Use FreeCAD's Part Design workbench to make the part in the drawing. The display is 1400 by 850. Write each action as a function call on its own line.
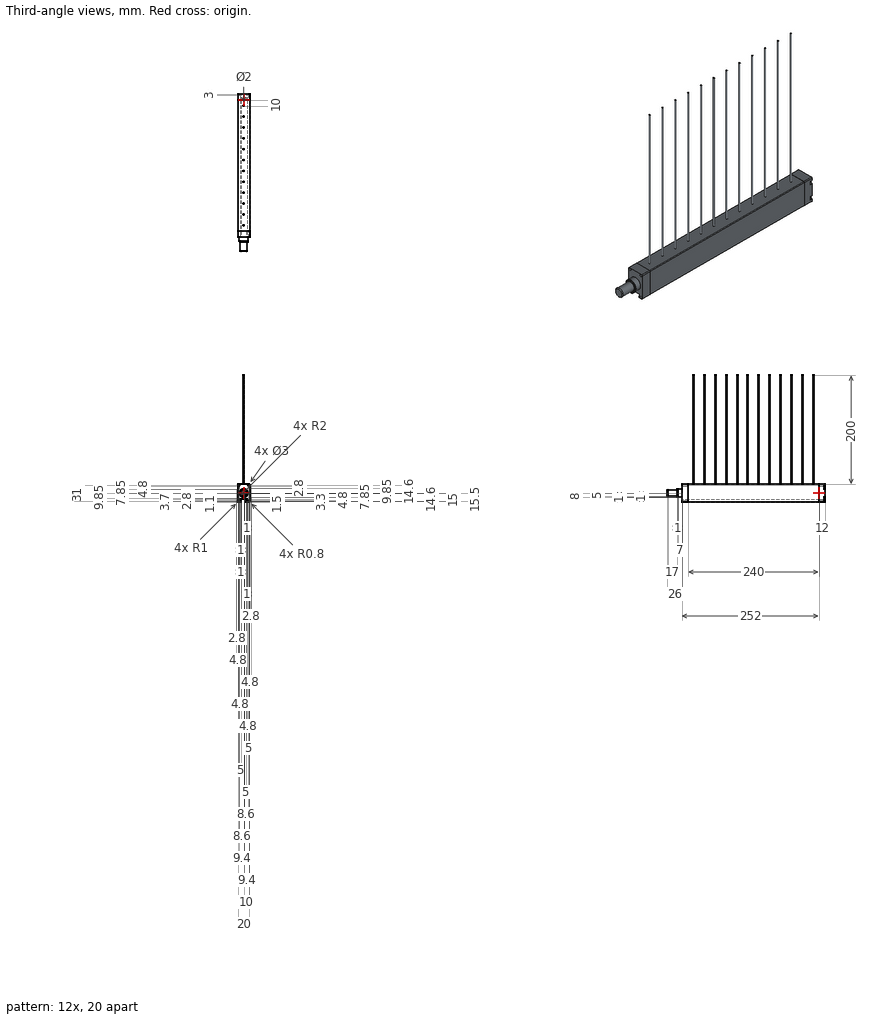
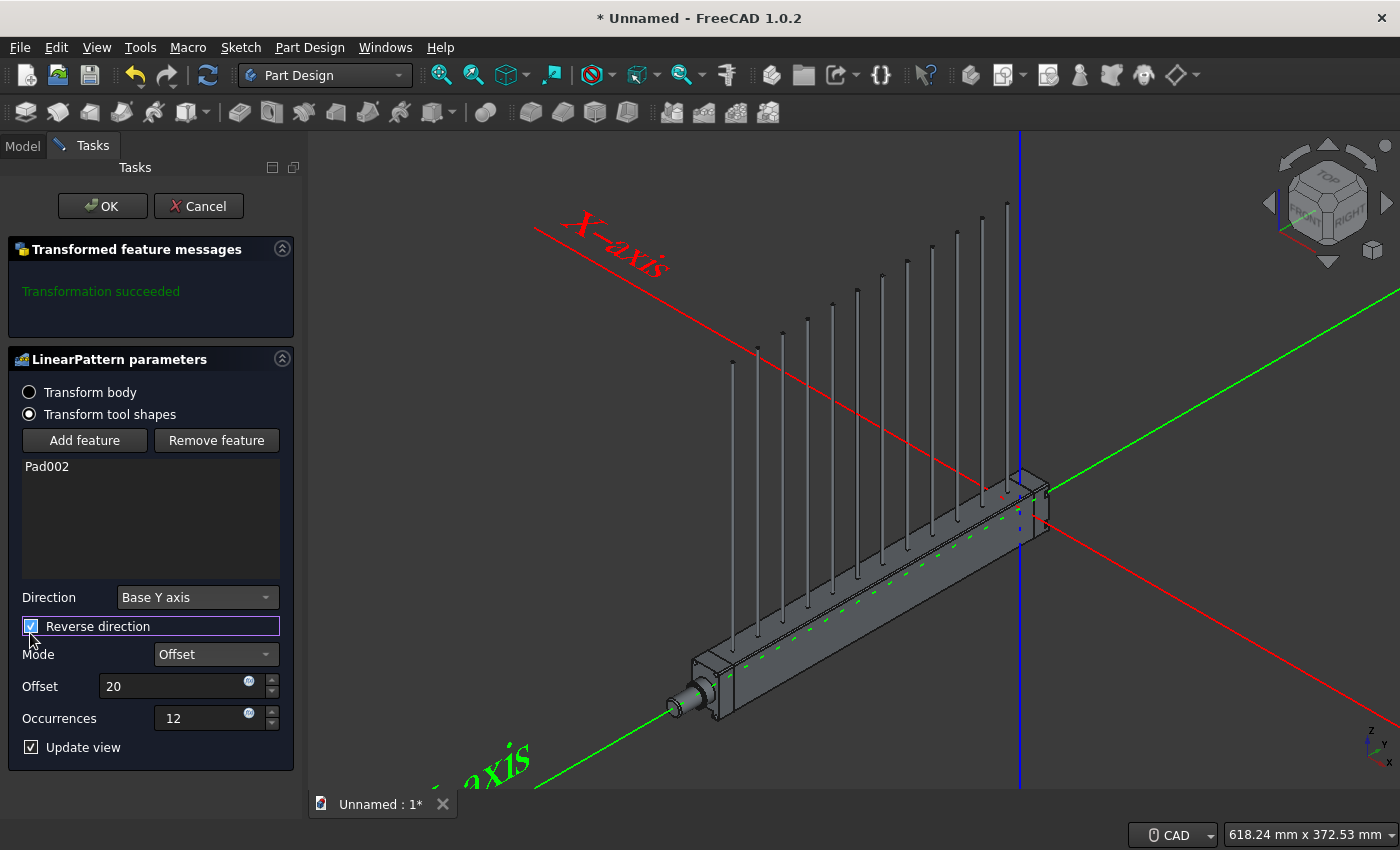
click(103, 206)